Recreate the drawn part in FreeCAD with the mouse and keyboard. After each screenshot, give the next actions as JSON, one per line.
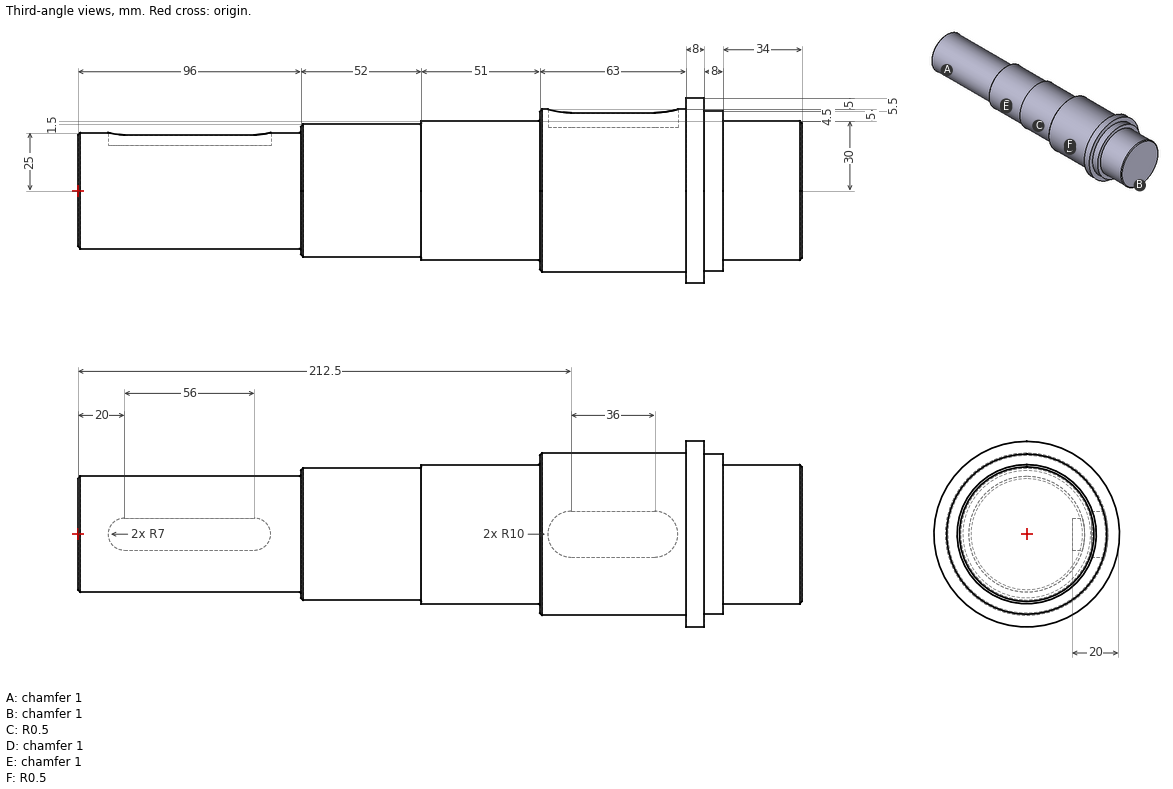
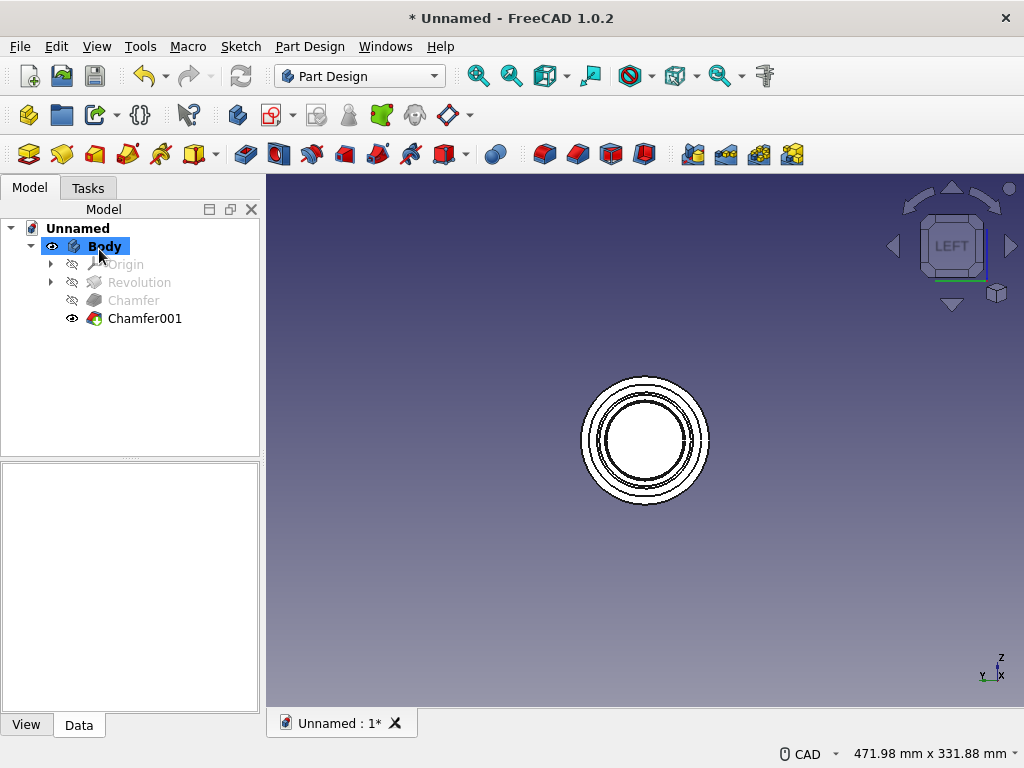
{"action": "key", "text": "v f"}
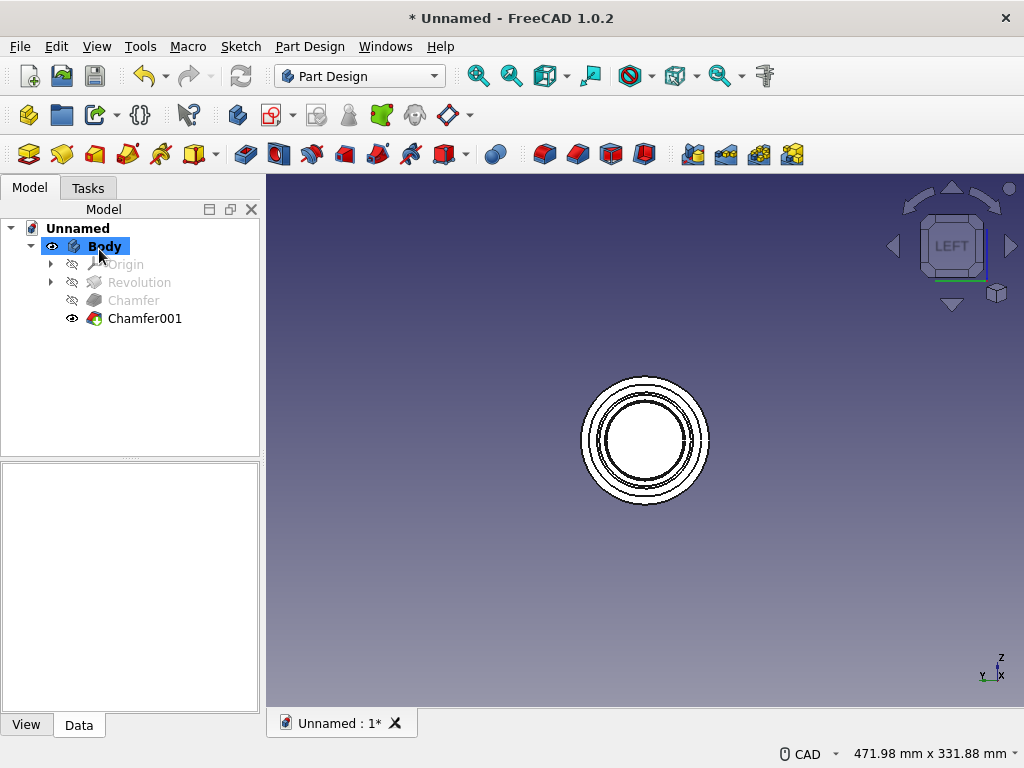
{"action": "key", "text": "v 3"}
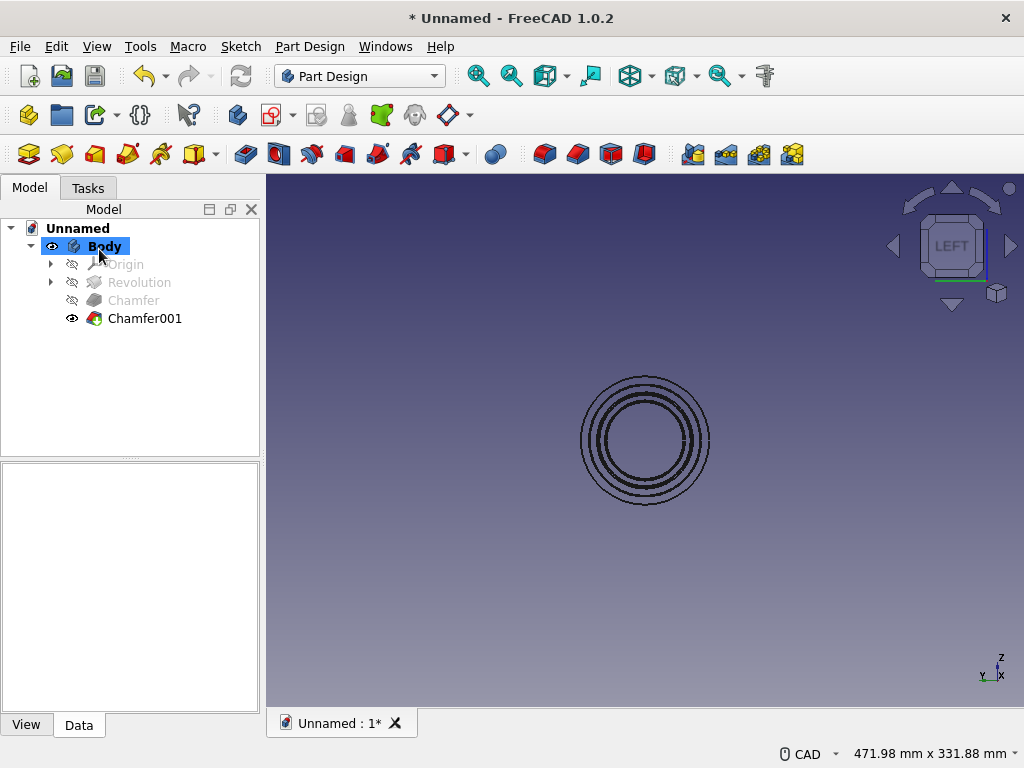
{"action": "key", "text": "0"}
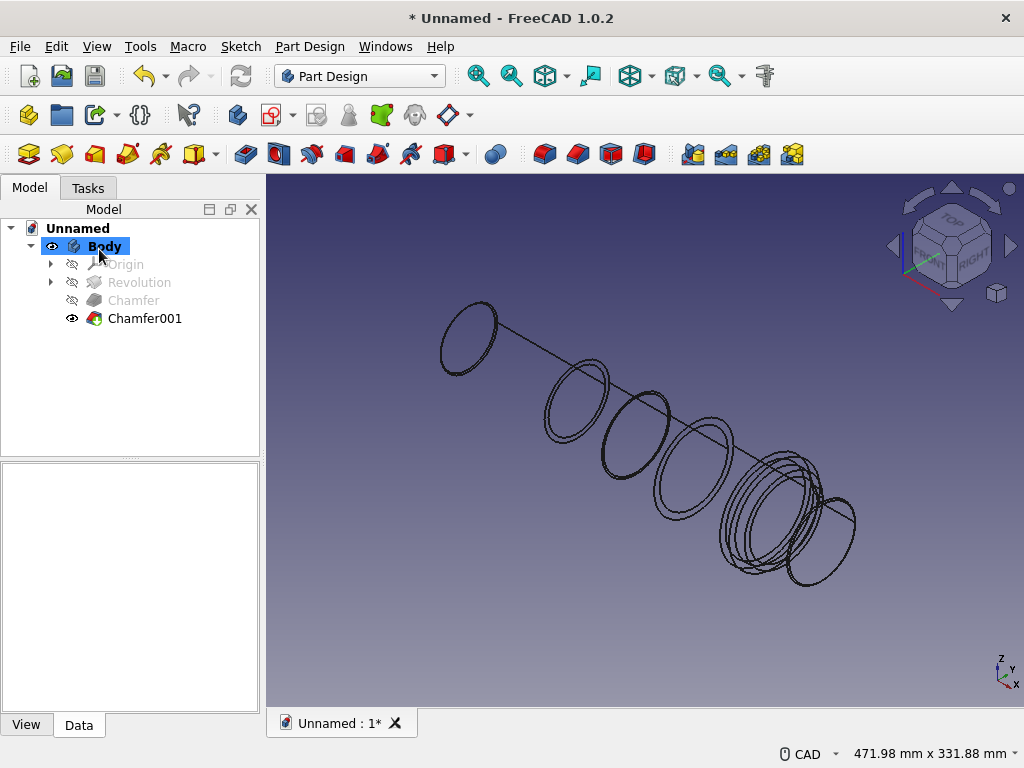
{"action": "left_click", "coordinate": [626, 476]}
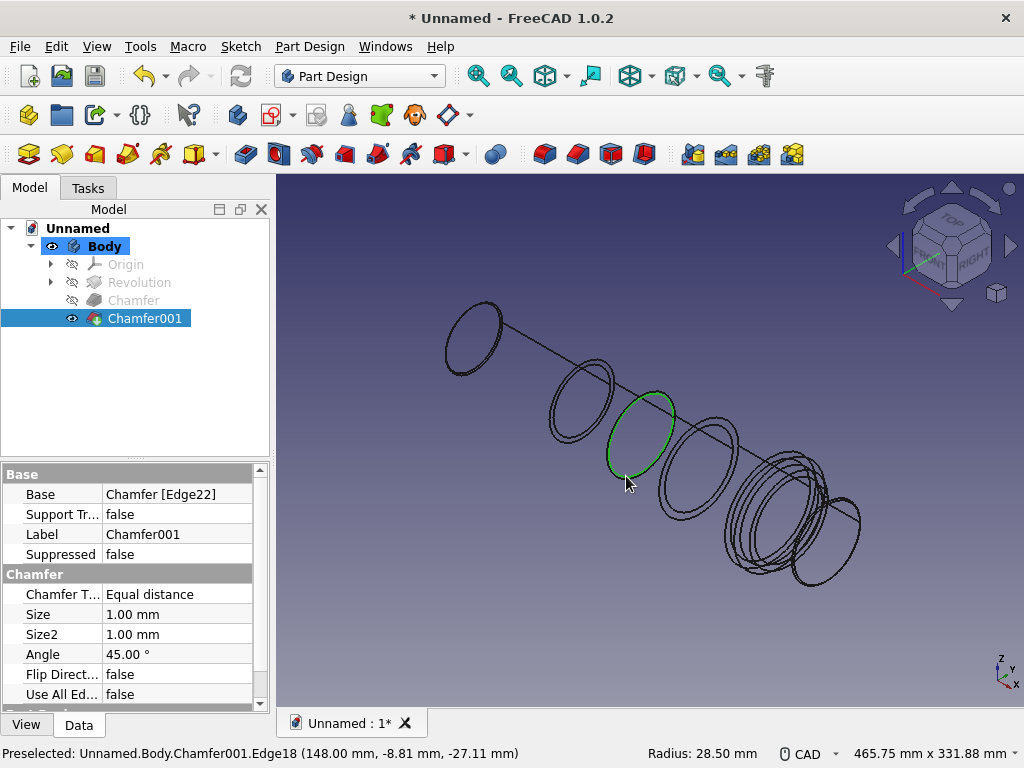
{"action": "left_click", "coordinate": [573, 436], "text": "ctrl"}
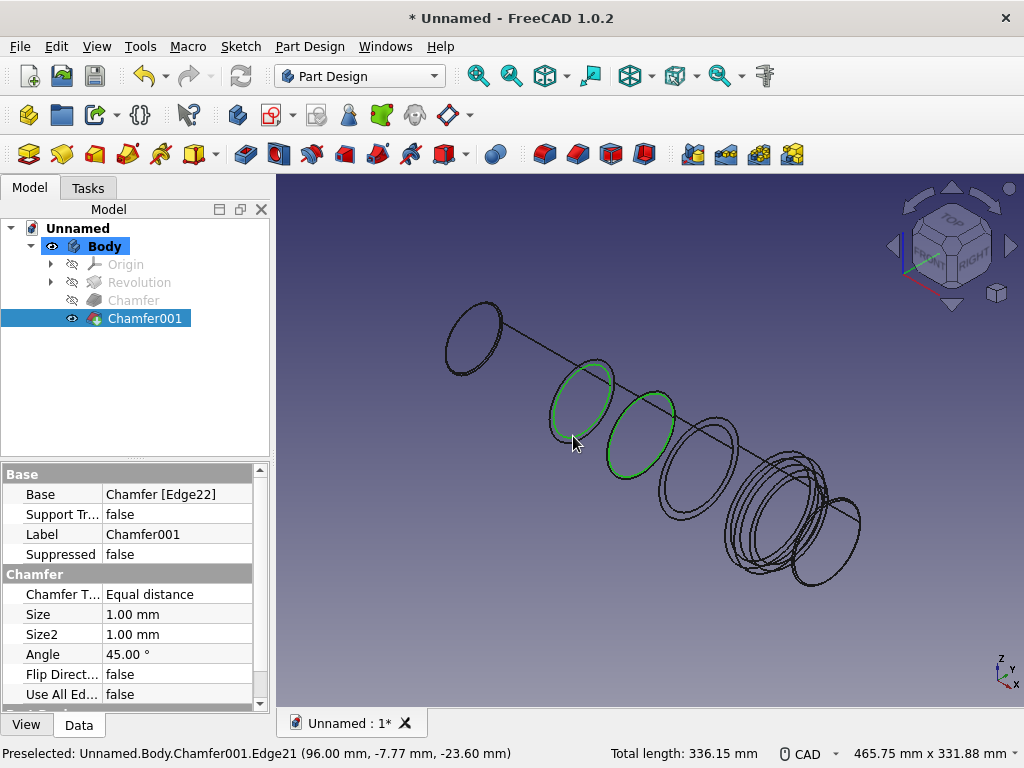
{"action": "key", "text": "v 1"}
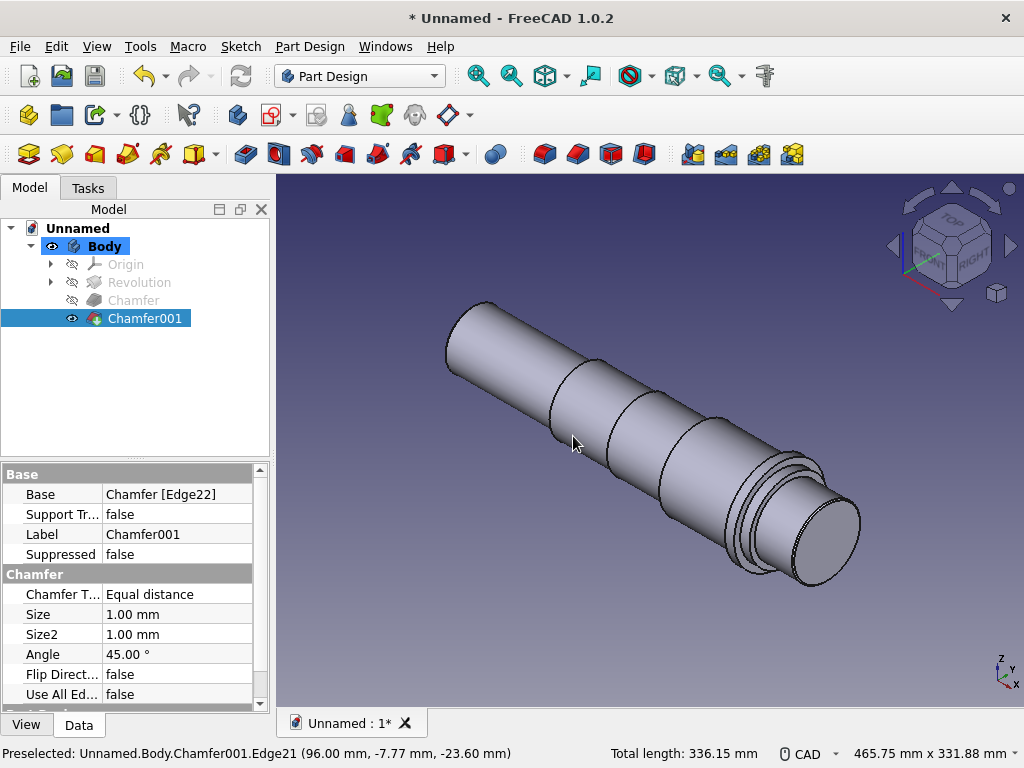
{"action": "left_click", "coordinate": [545, 154]}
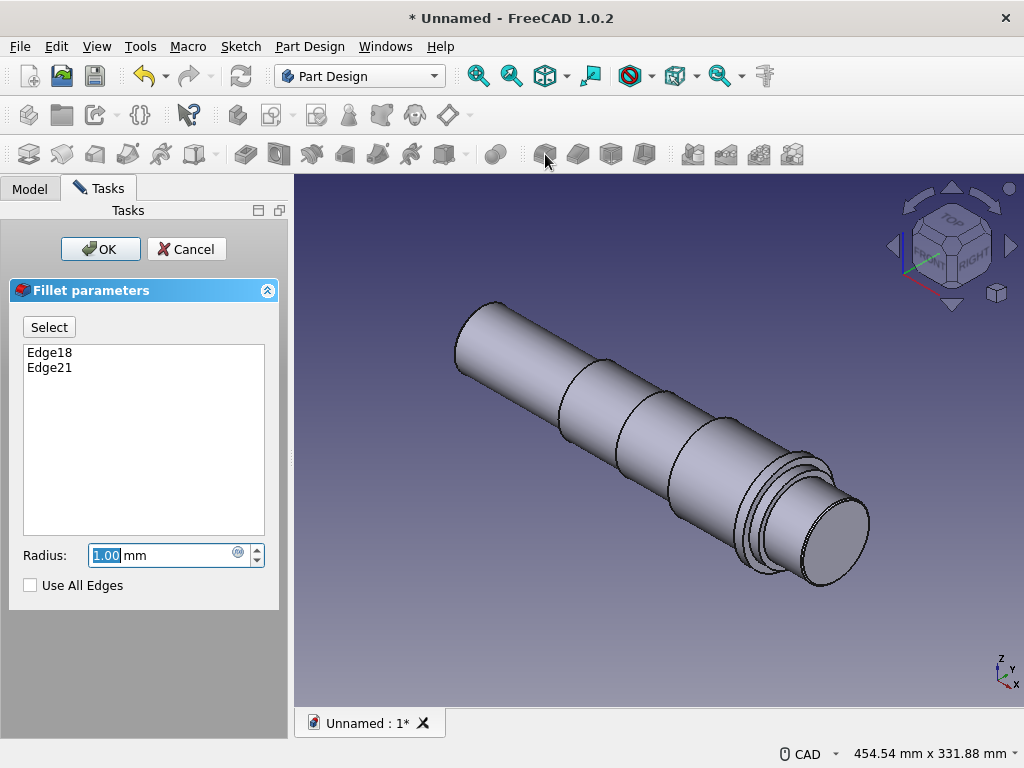
{"action": "type", "text": "0.5"}
{"action": "key", "text": "Tab"}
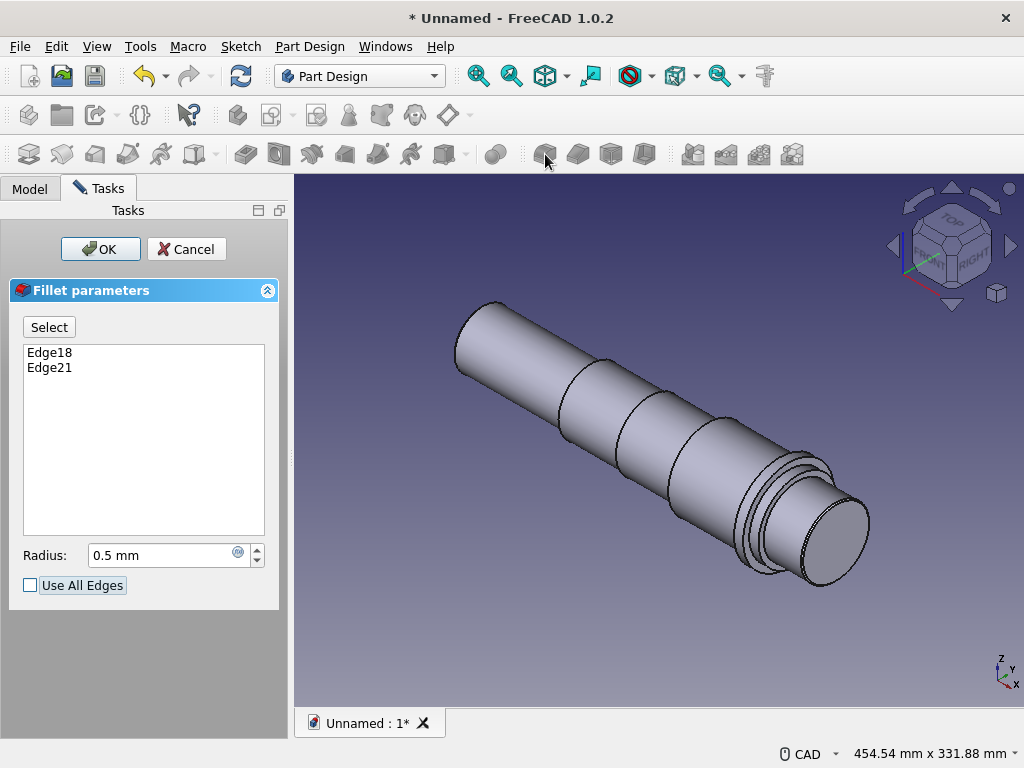
{"action": "left_click", "coordinate": [101, 249]}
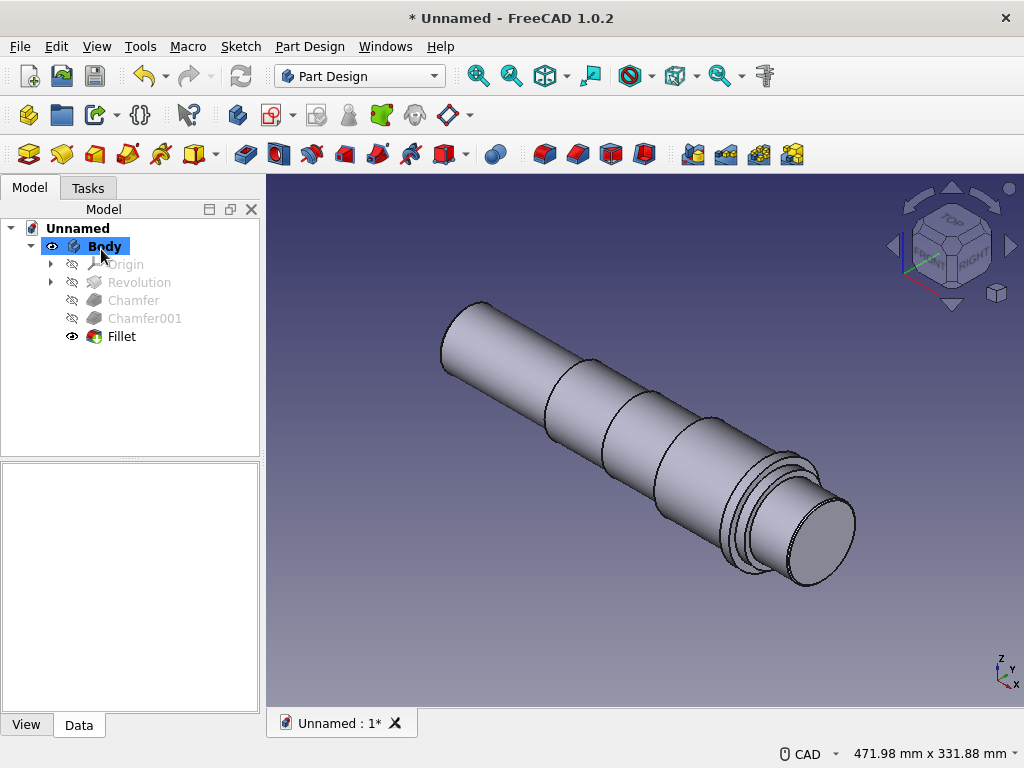
{"action": "key", "text": "2"}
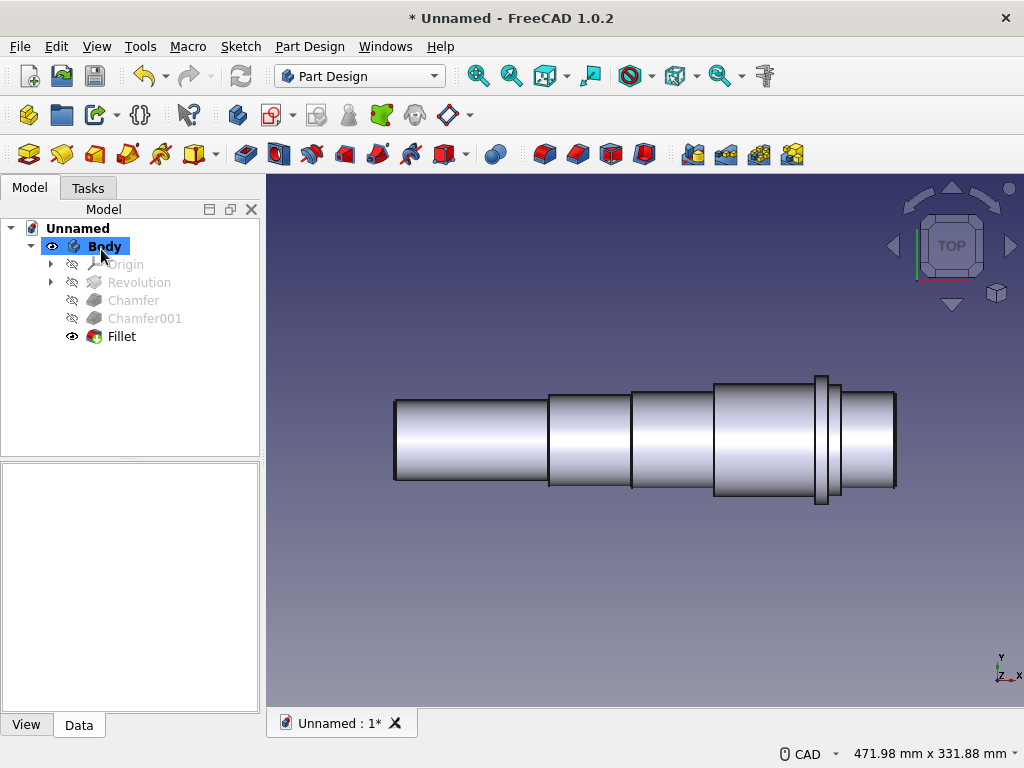
{"action": "left_click", "coordinate": [714, 485]}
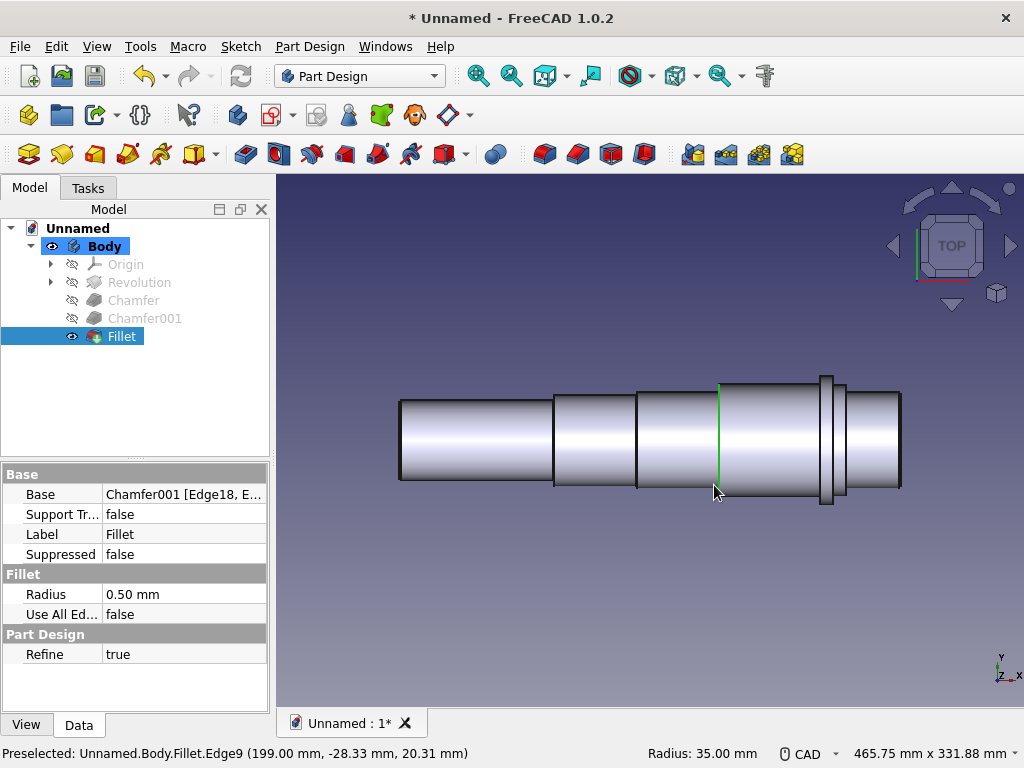
{"action": "left_click", "coordinate": [578, 154]}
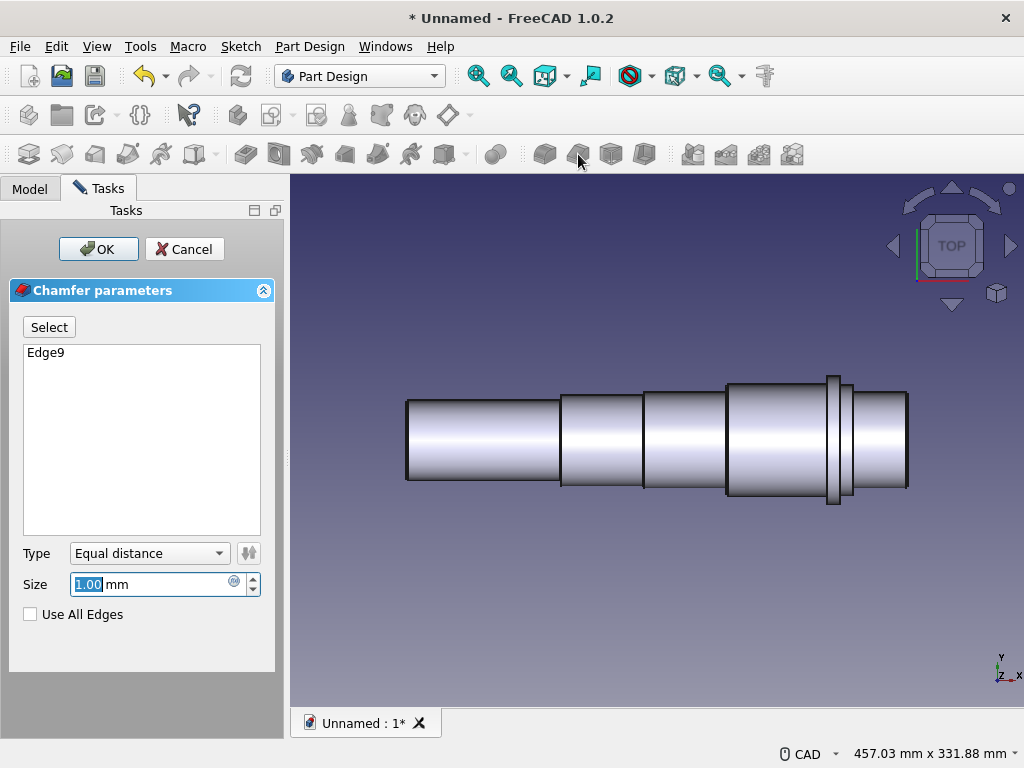
{"action": "type", "text": "1"}
{"action": "key", "text": "Tab"}